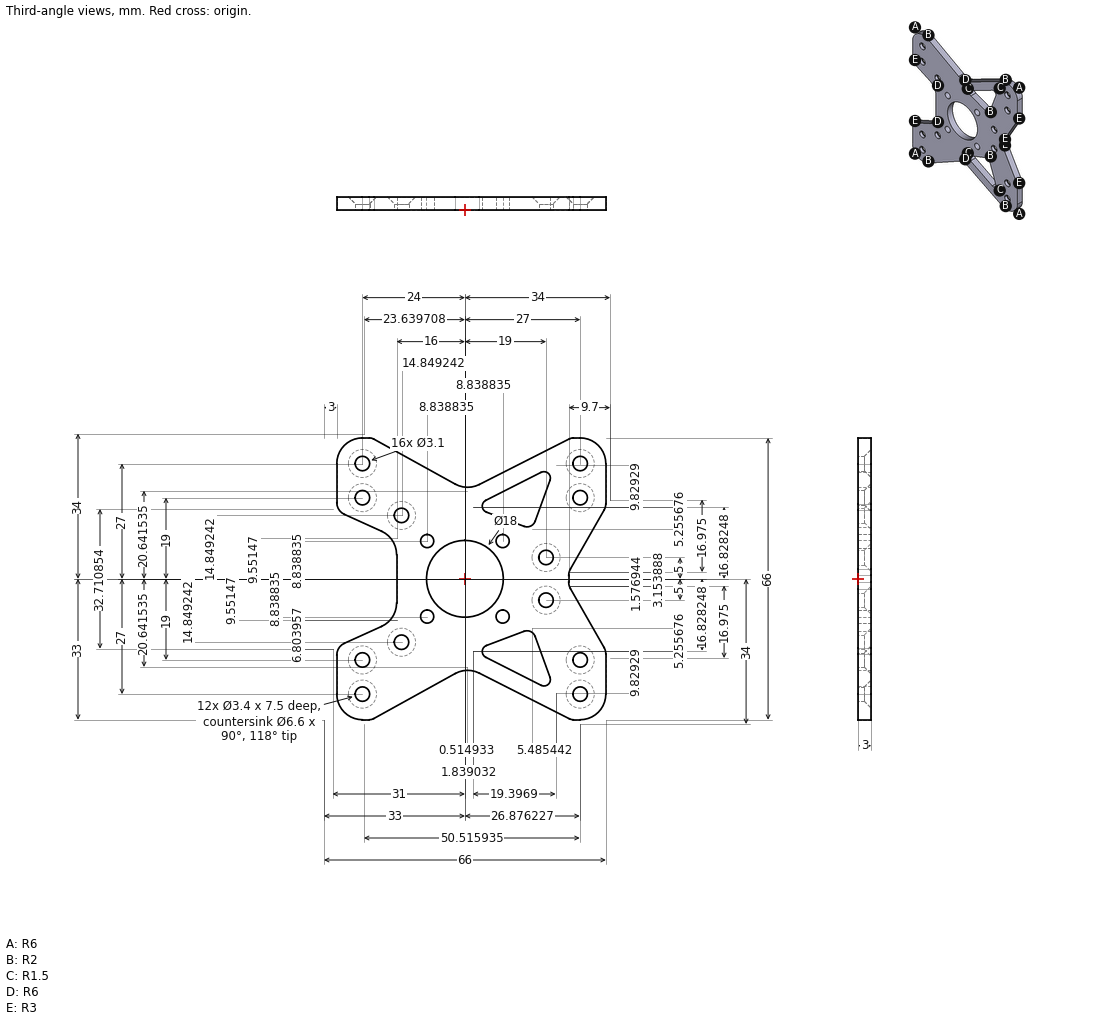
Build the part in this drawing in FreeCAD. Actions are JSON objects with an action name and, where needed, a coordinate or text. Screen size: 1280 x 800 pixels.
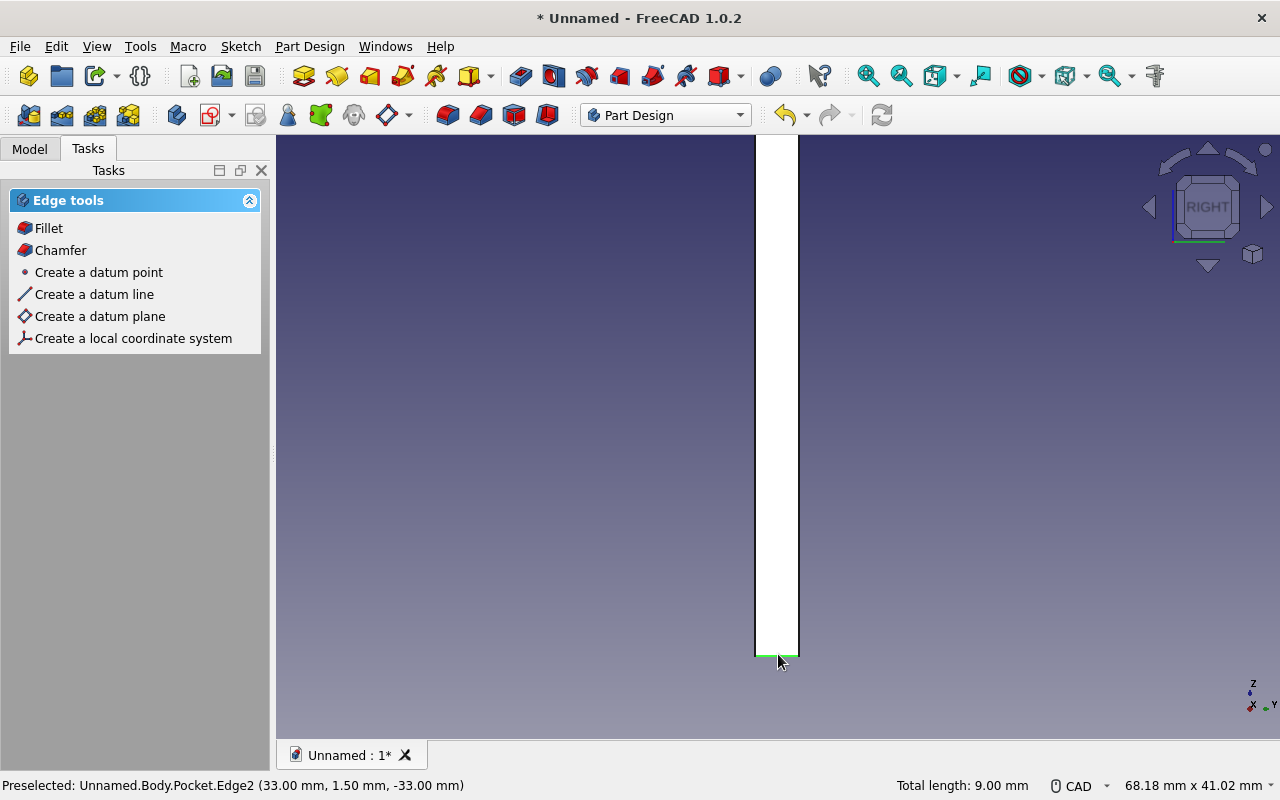
{"action": "left_click", "coordinate": [869, 76]}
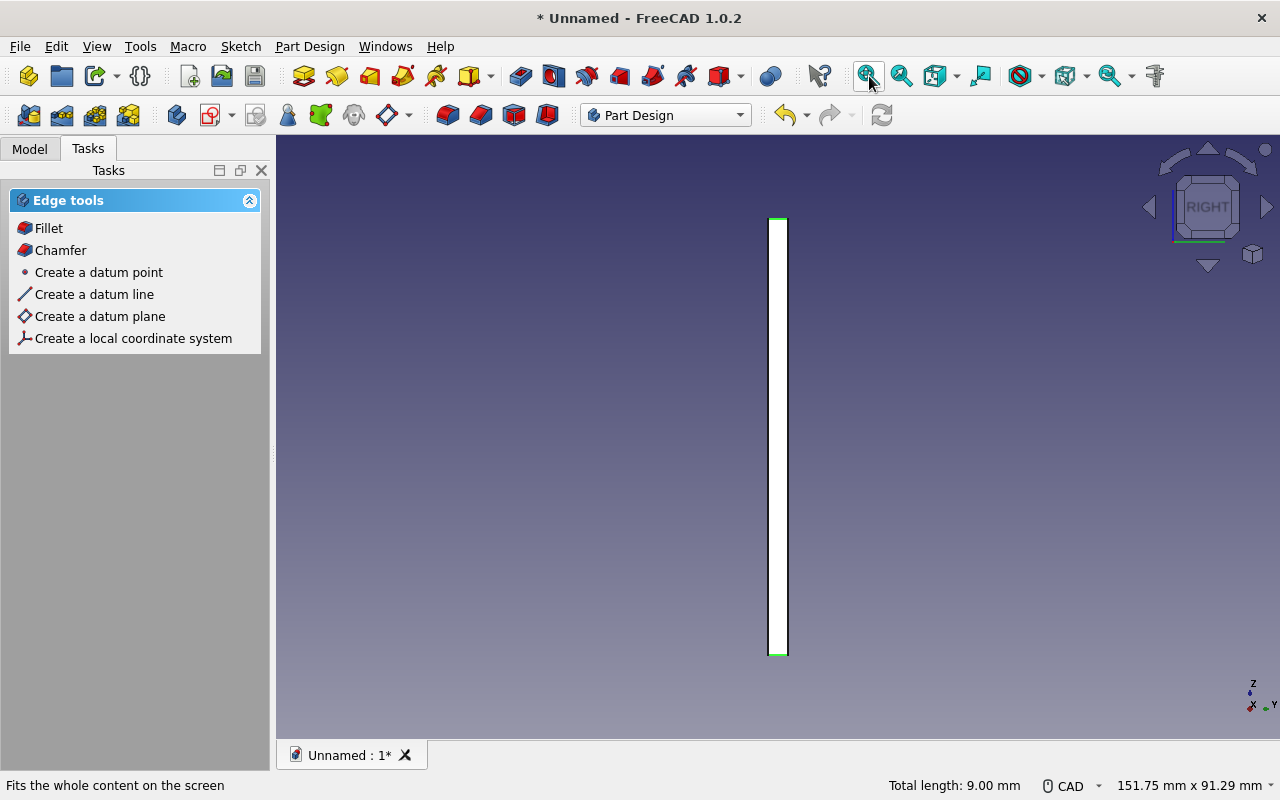
{"action": "key", "text": "5"}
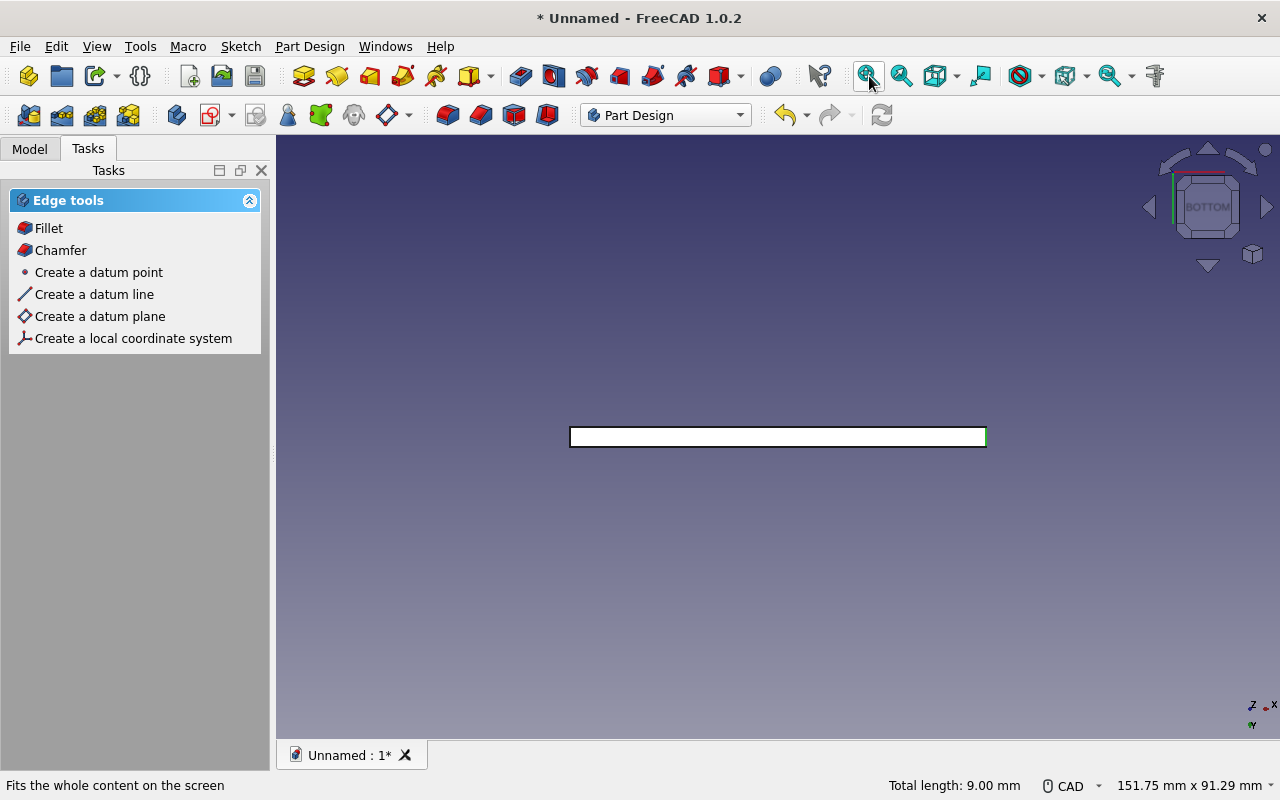
{"action": "left_click", "coordinate": [869, 76]}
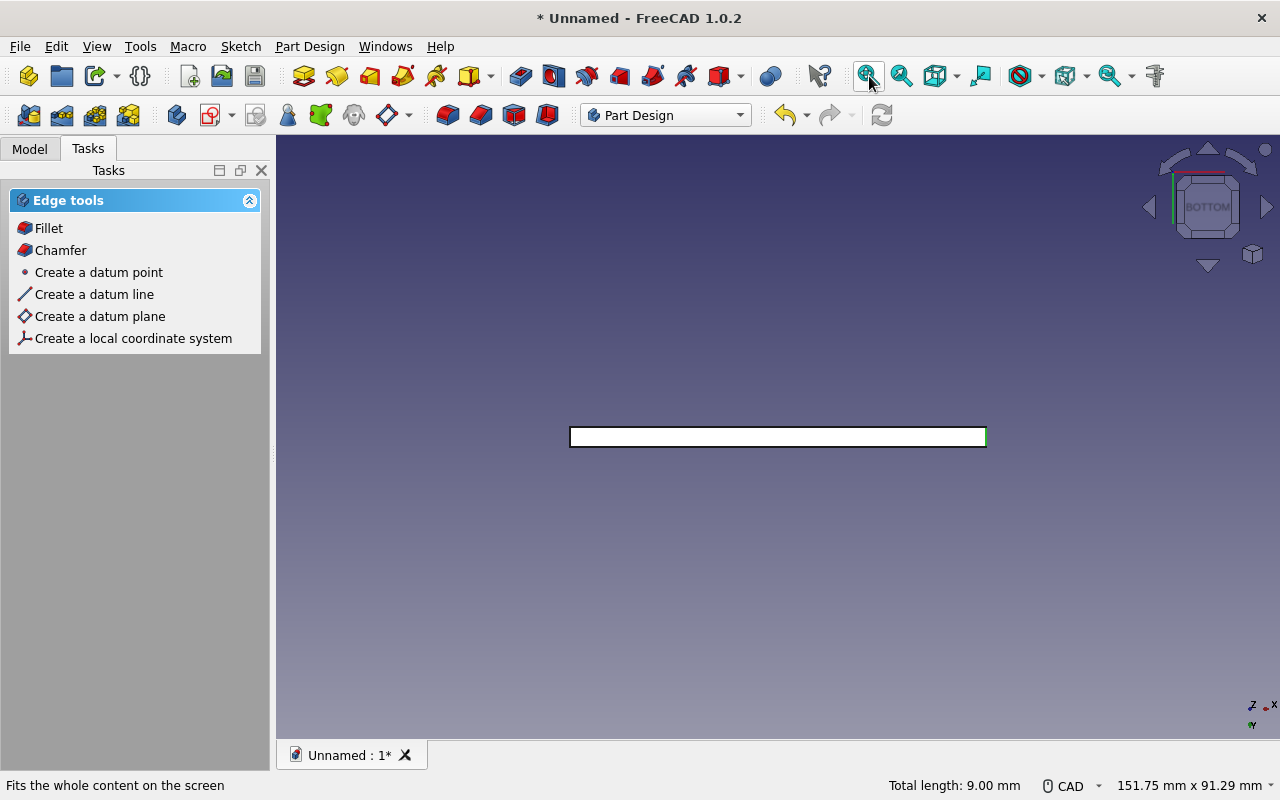
{"action": "left_click", "coordinate": [570, 436], "text": "ctrl"}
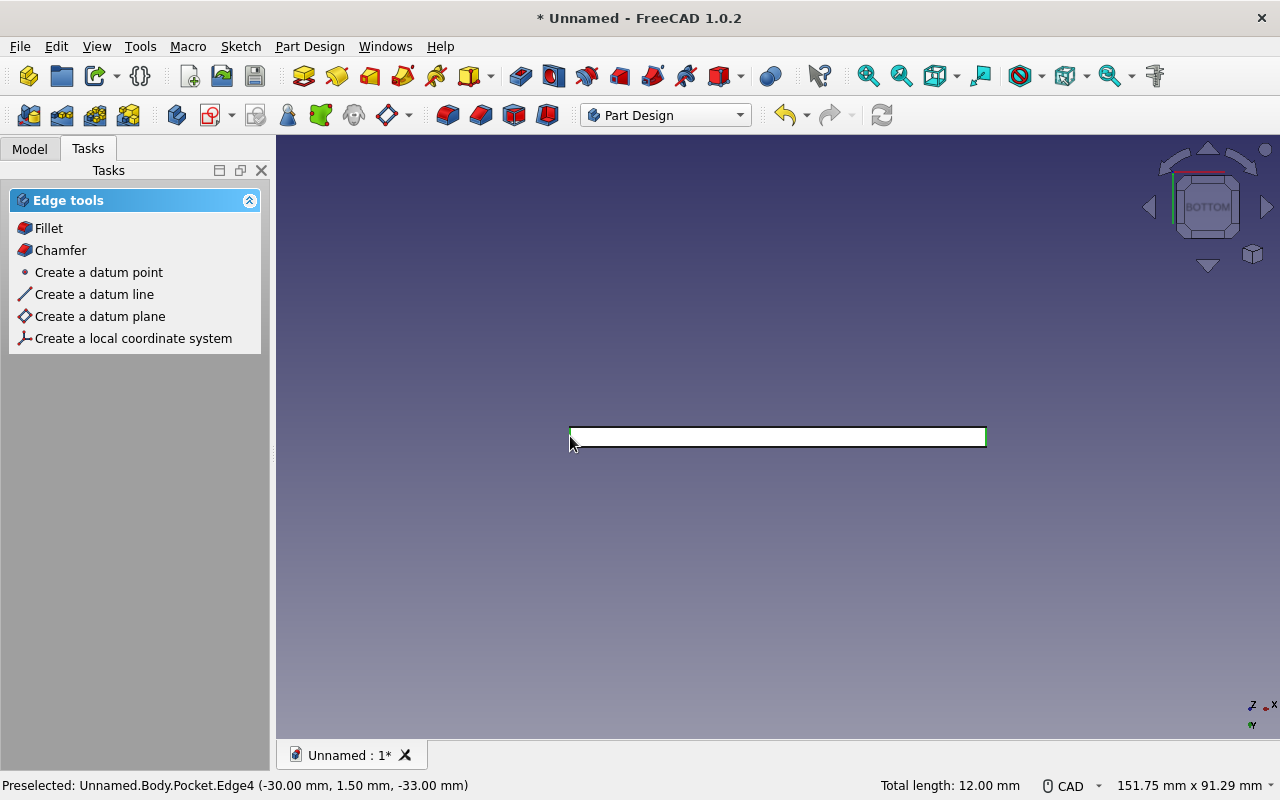
{"action": "left_click", "coordinate": [448, 116]}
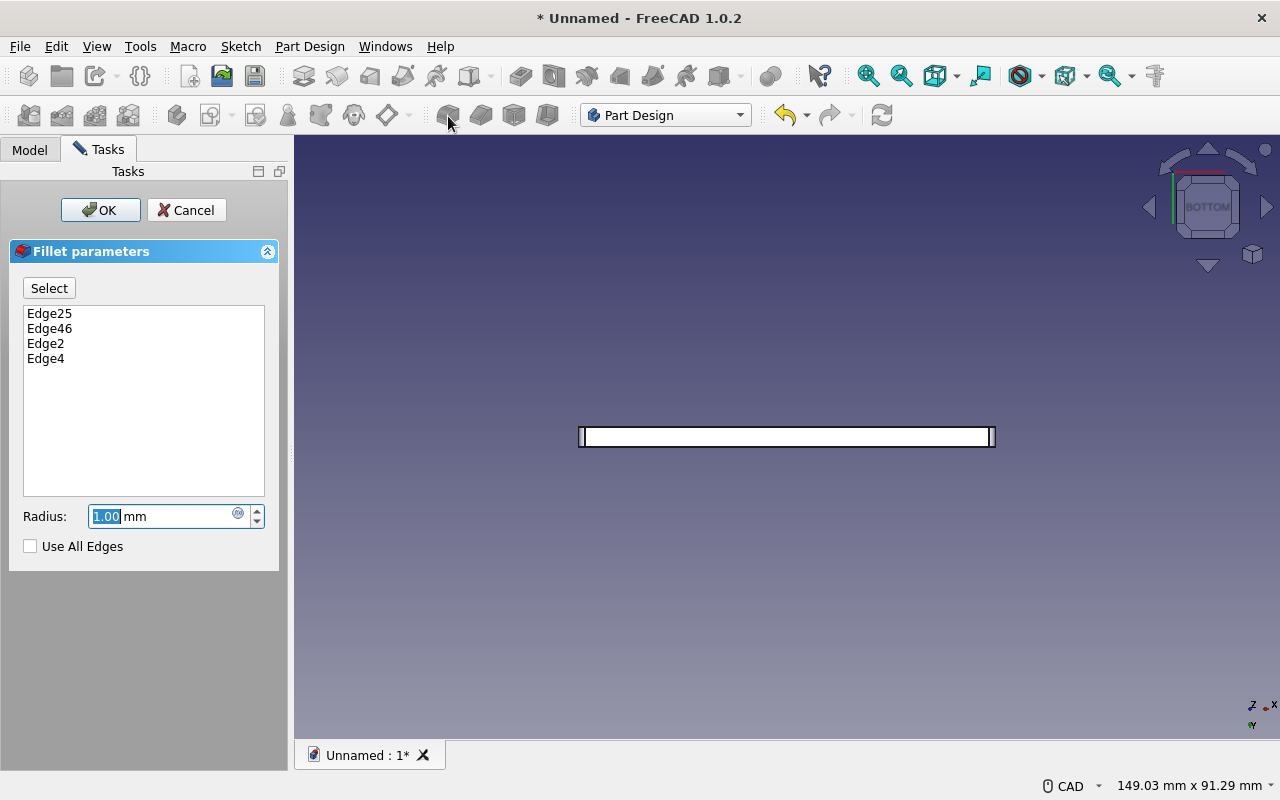
{"action": "type", "text": "6"}
{"action": "key", "text": "Tab"}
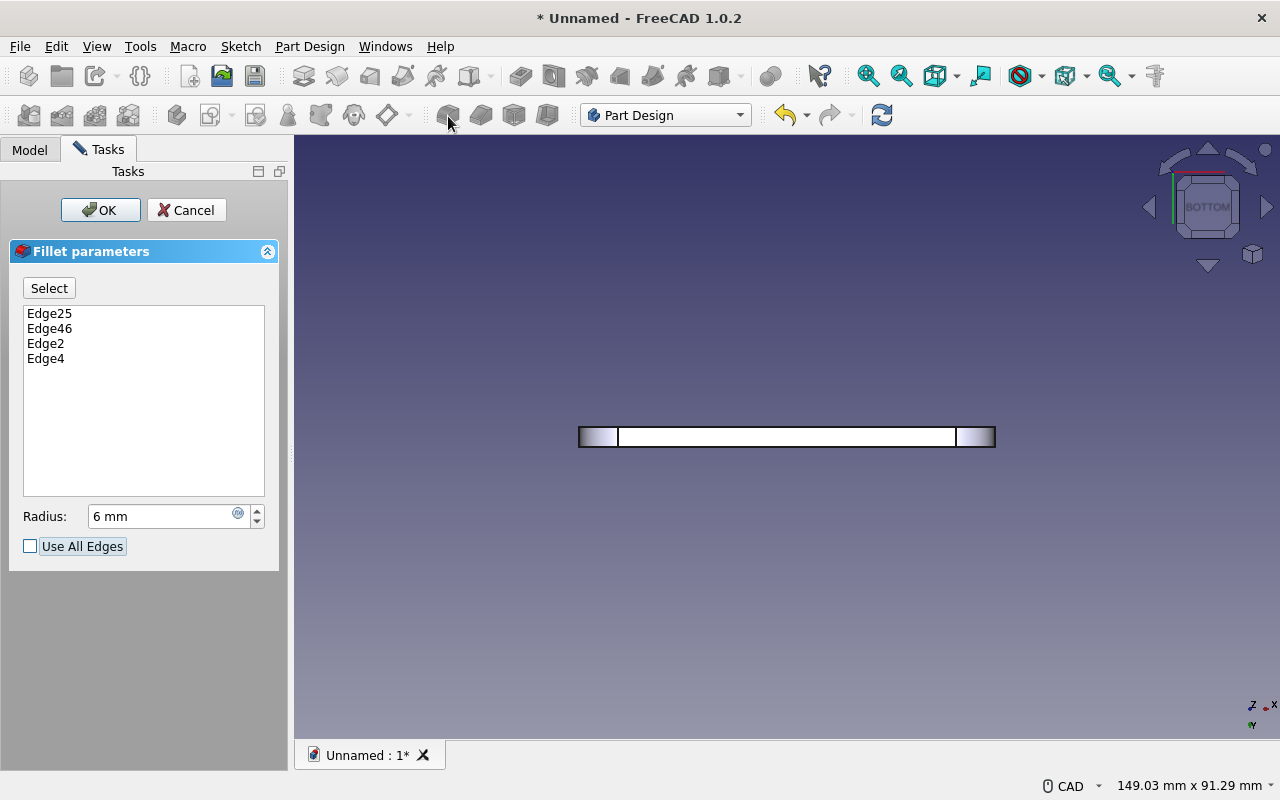
{"action": "left_click", "coordinate": [101, 210]}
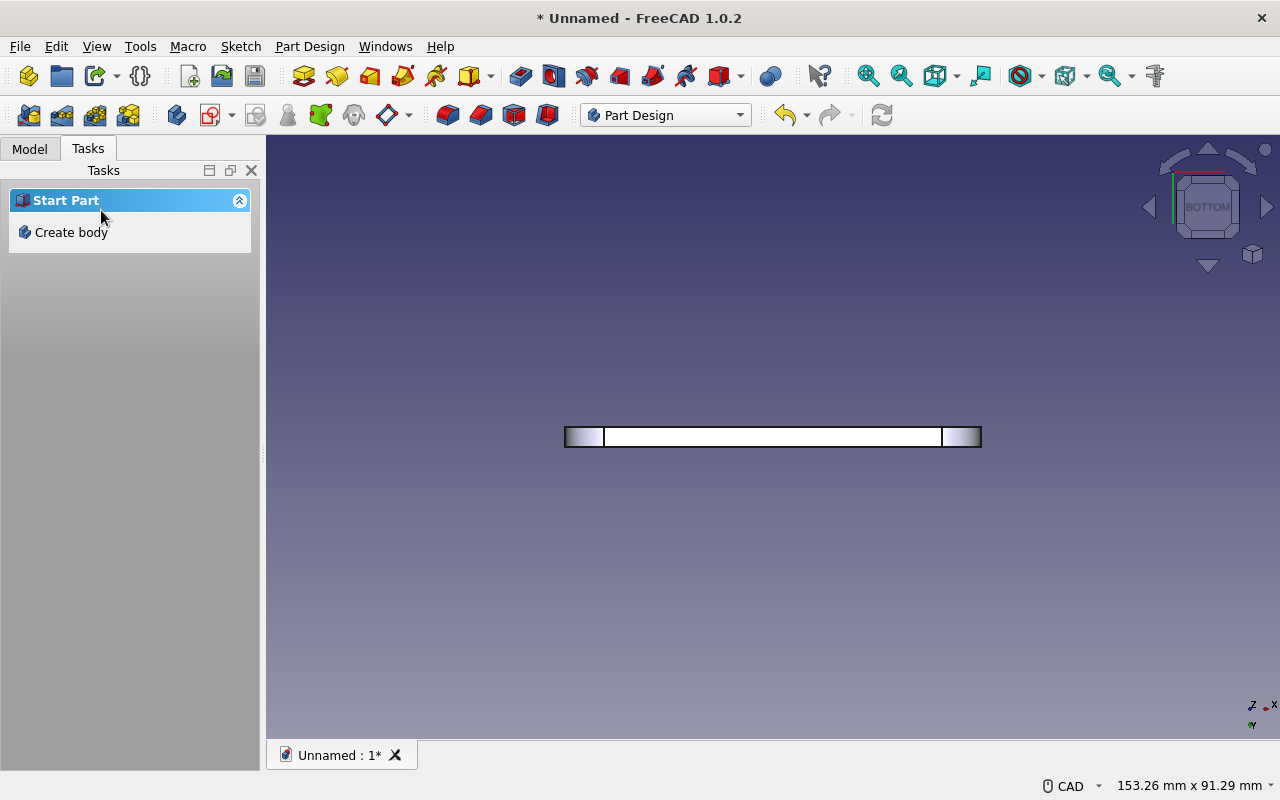
{"action": "left_click", "coordinate": [869, 76]}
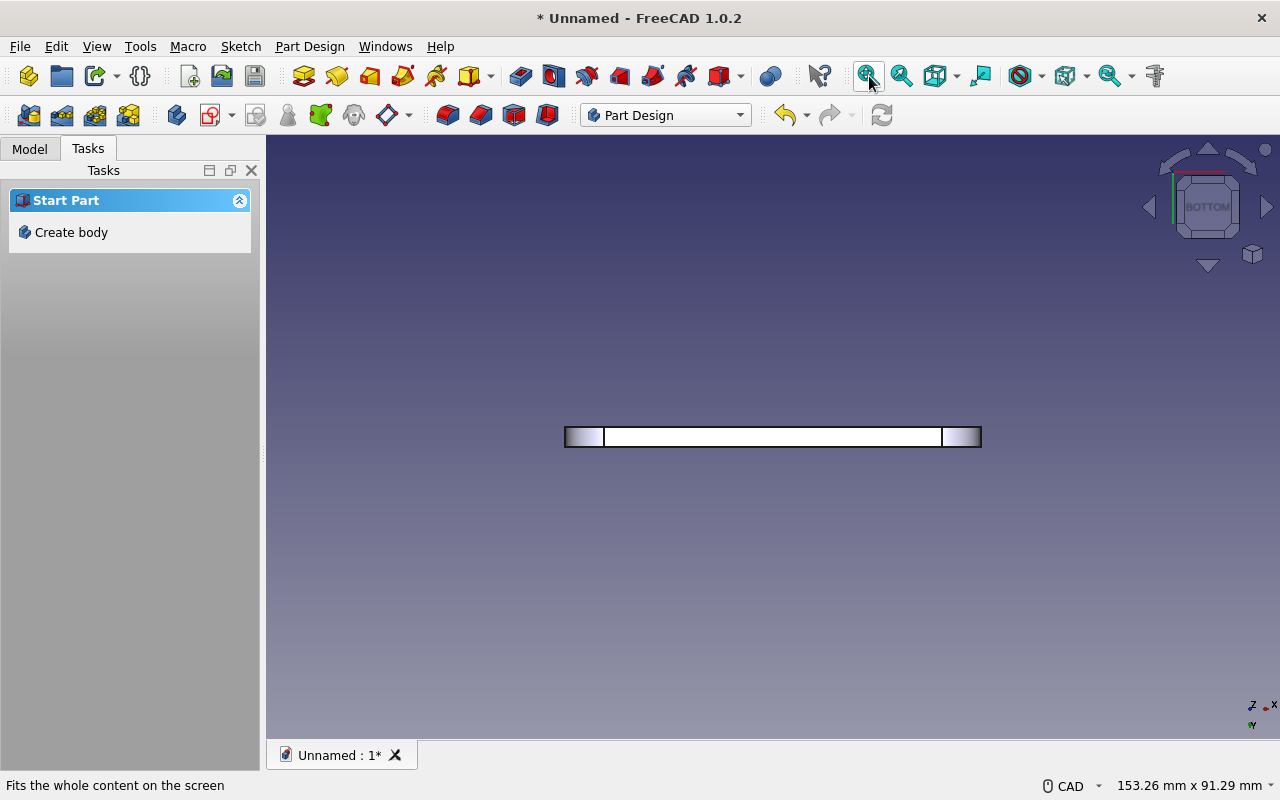
{"action": "key", "text": "4"}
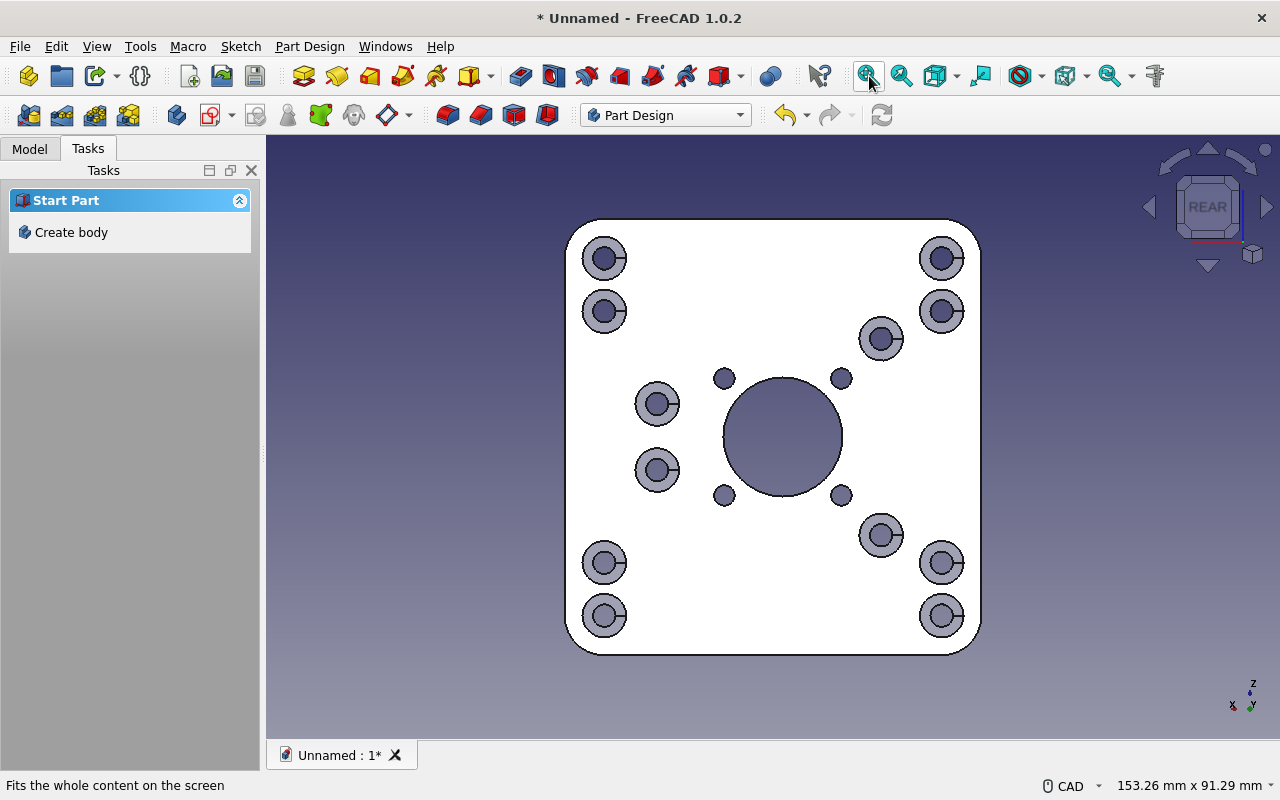
{"action": "left_click", "coordinate": [773, 561]}